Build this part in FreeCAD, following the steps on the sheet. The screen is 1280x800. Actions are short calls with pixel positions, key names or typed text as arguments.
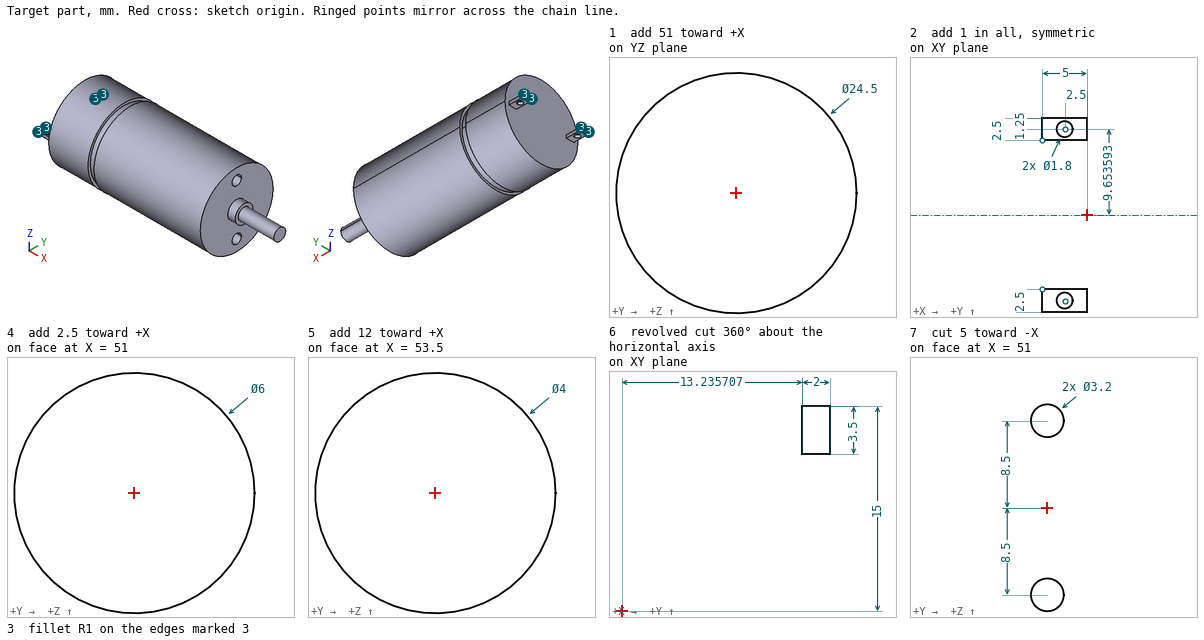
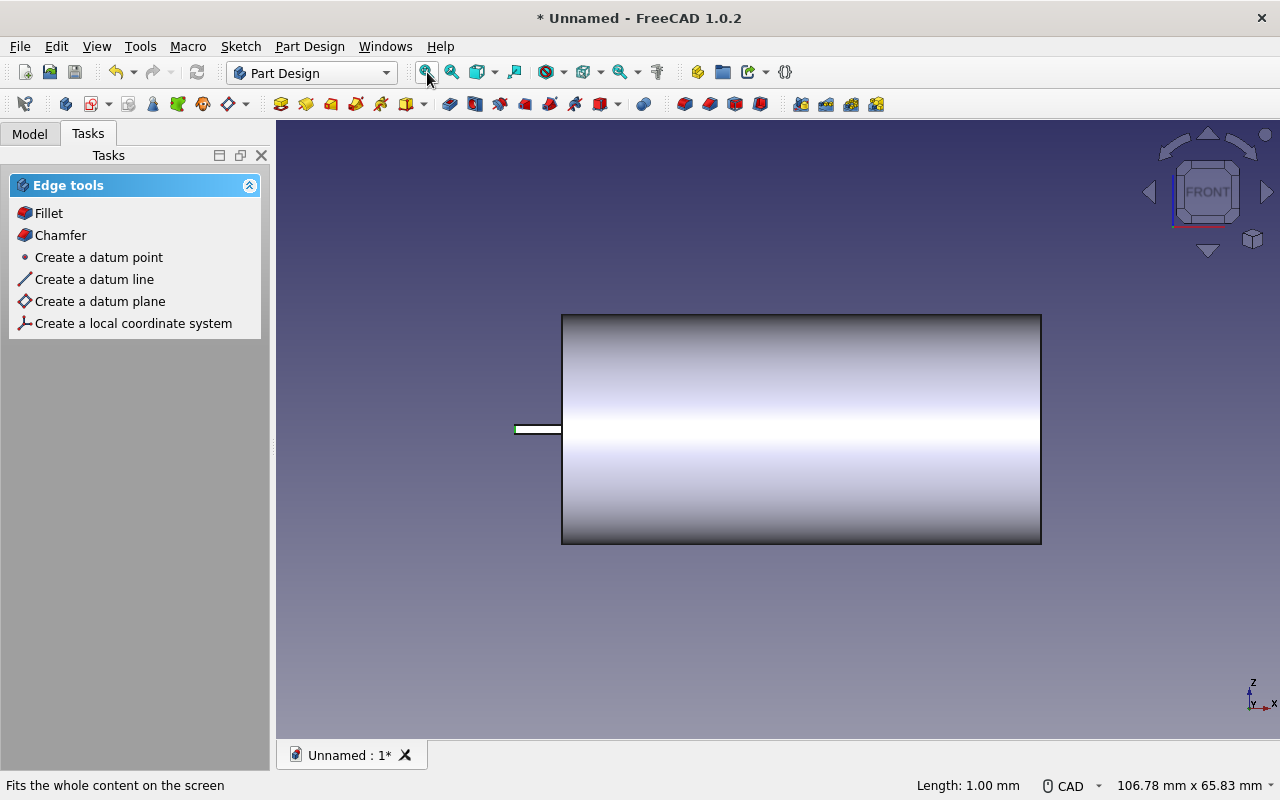
key(3)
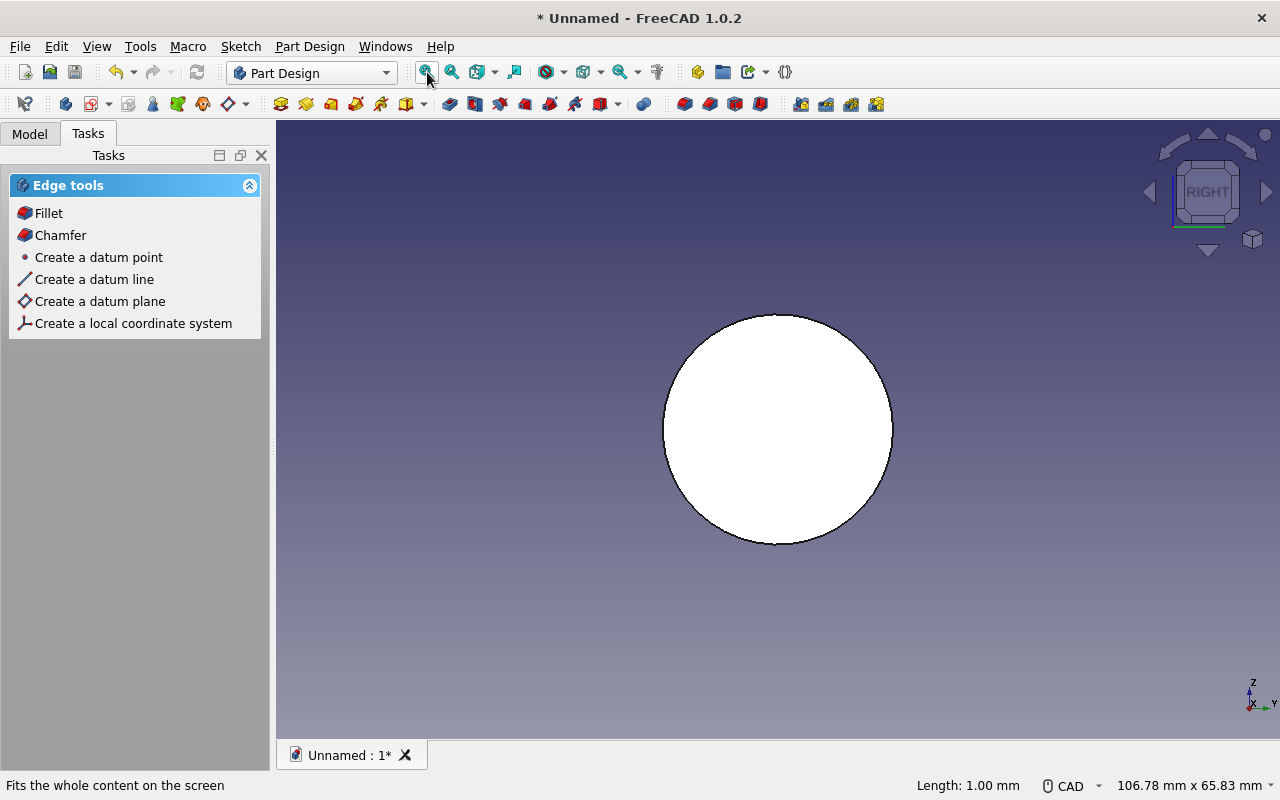
click(427, 72)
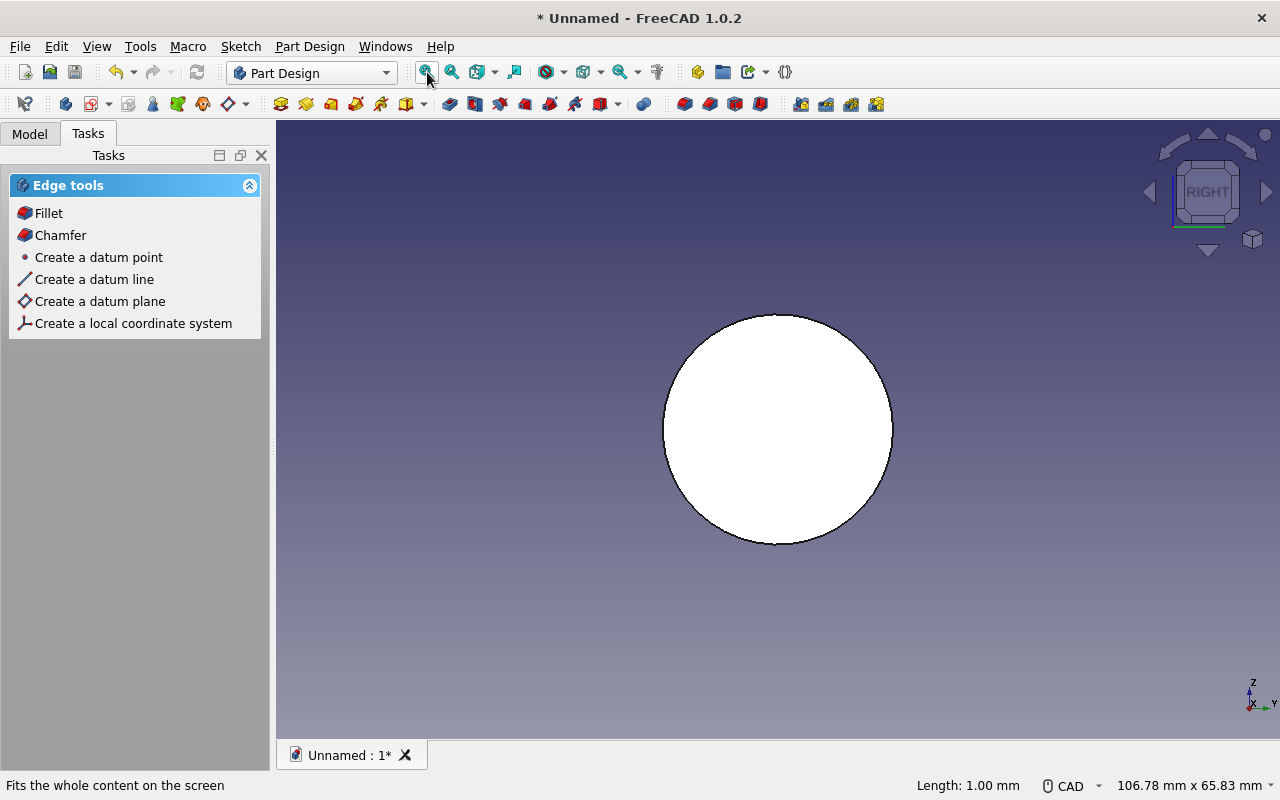
scroll(857, 428, up, 8)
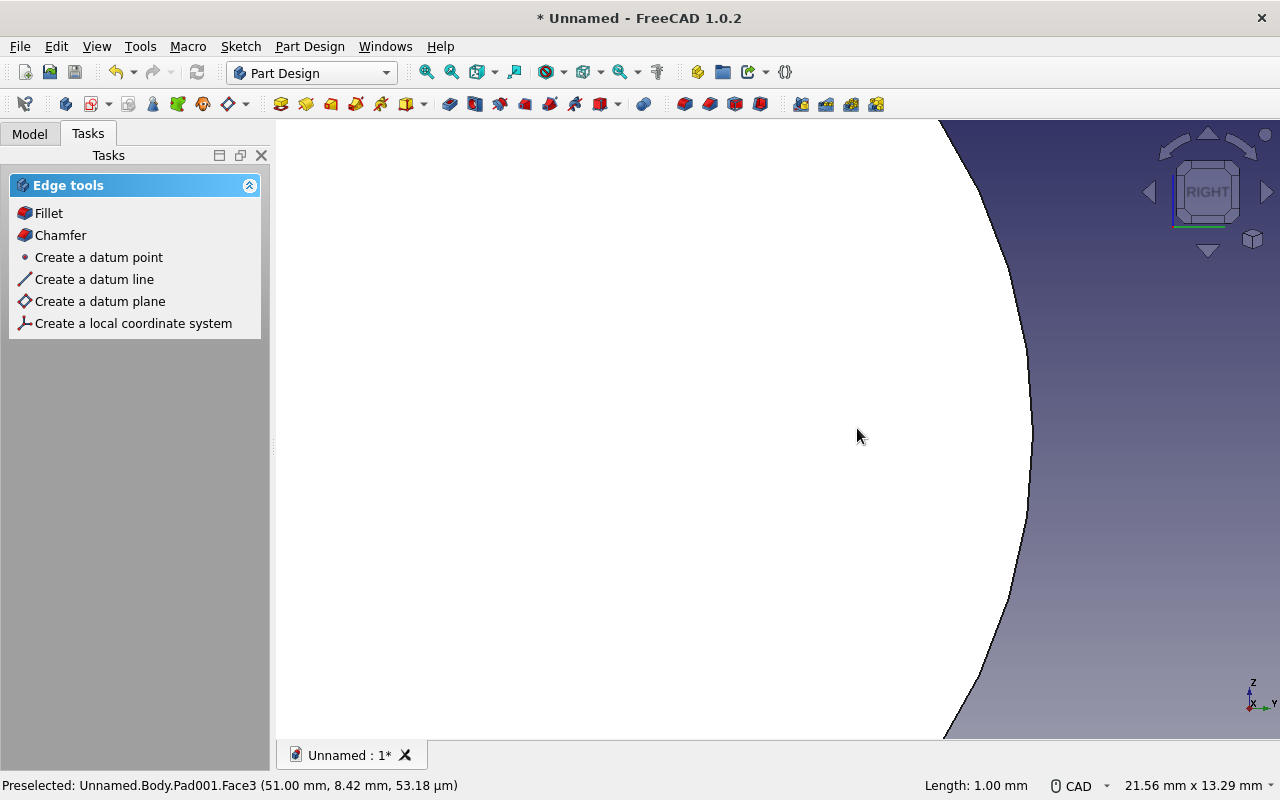
click(427, 72)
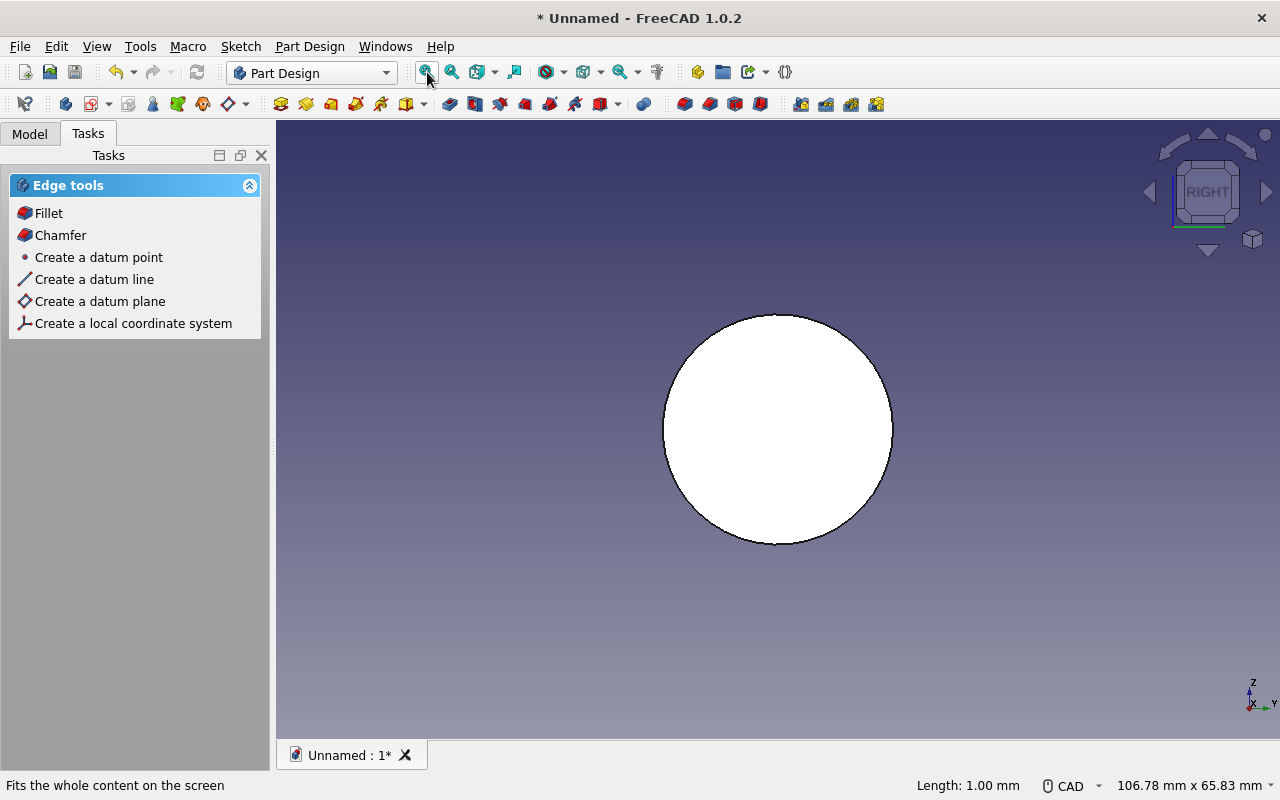
key(5)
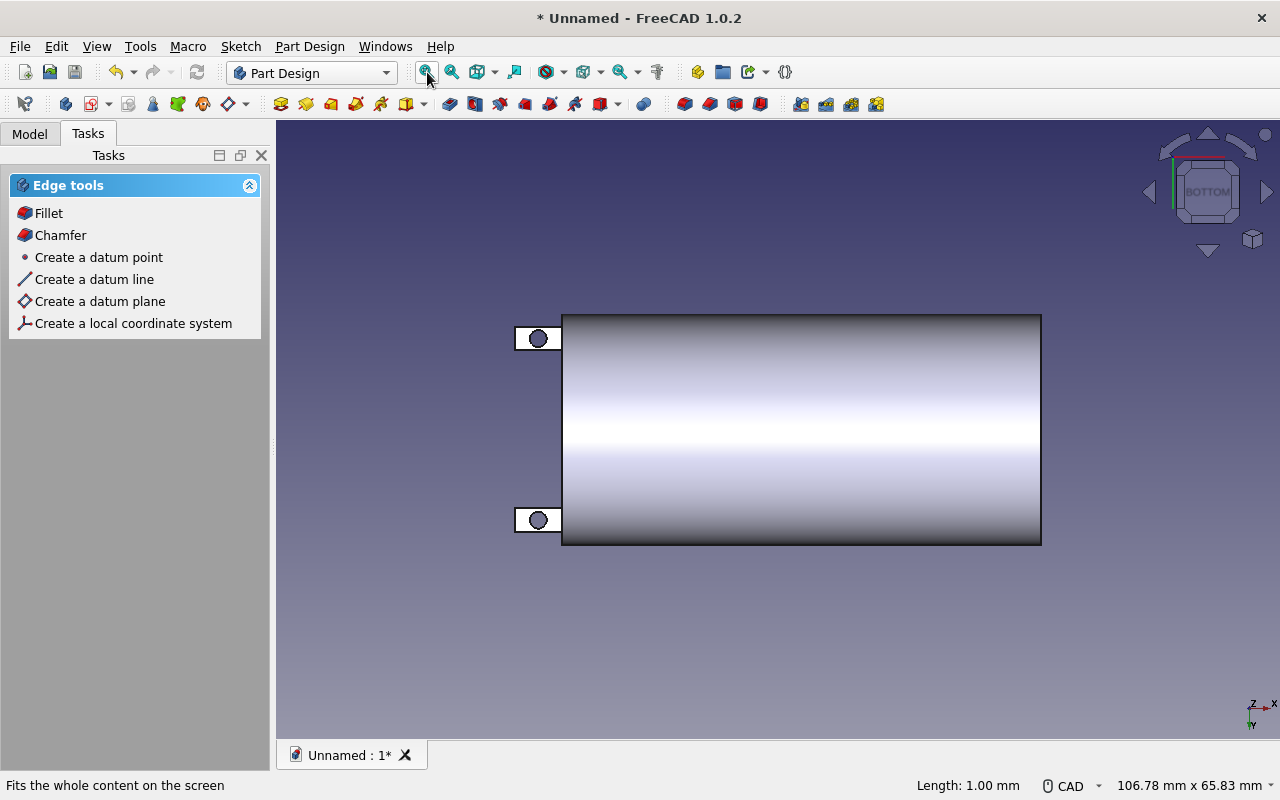
scroll(515, 507, up, 8)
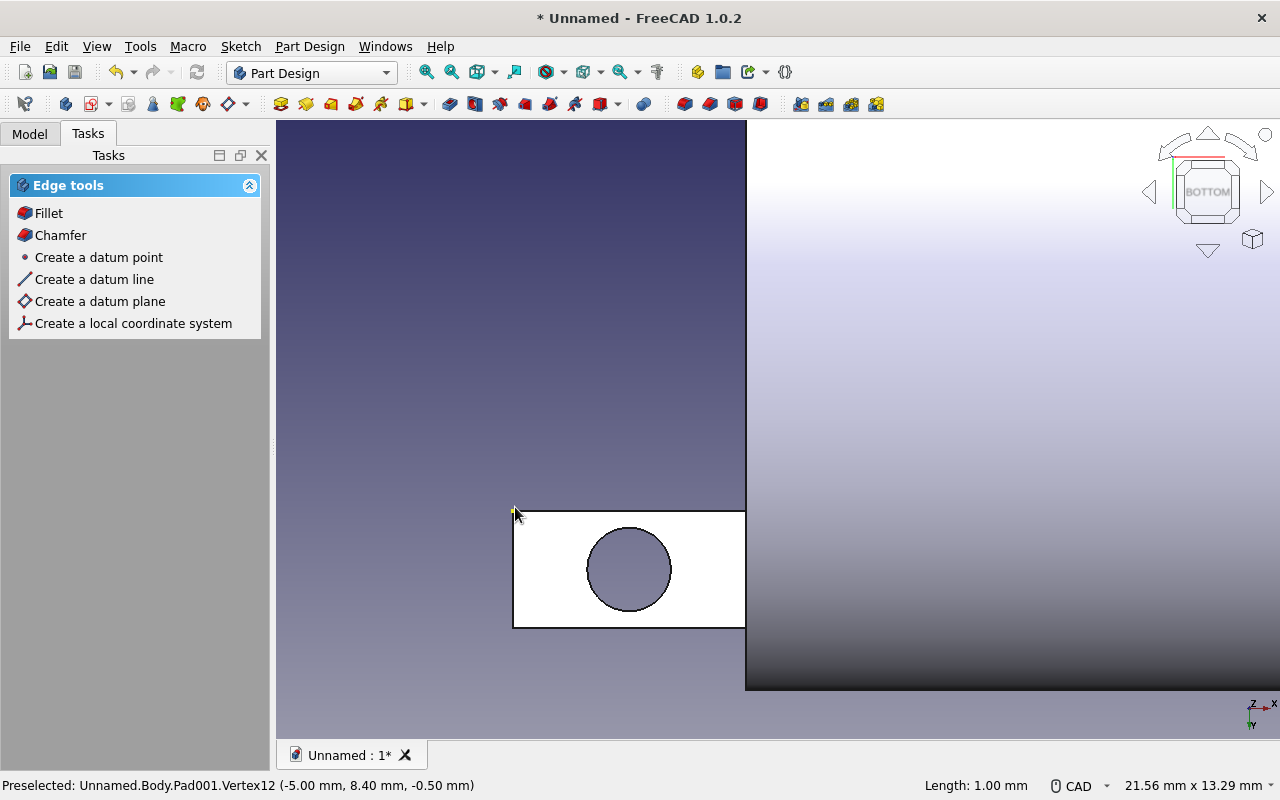
click(427, 72)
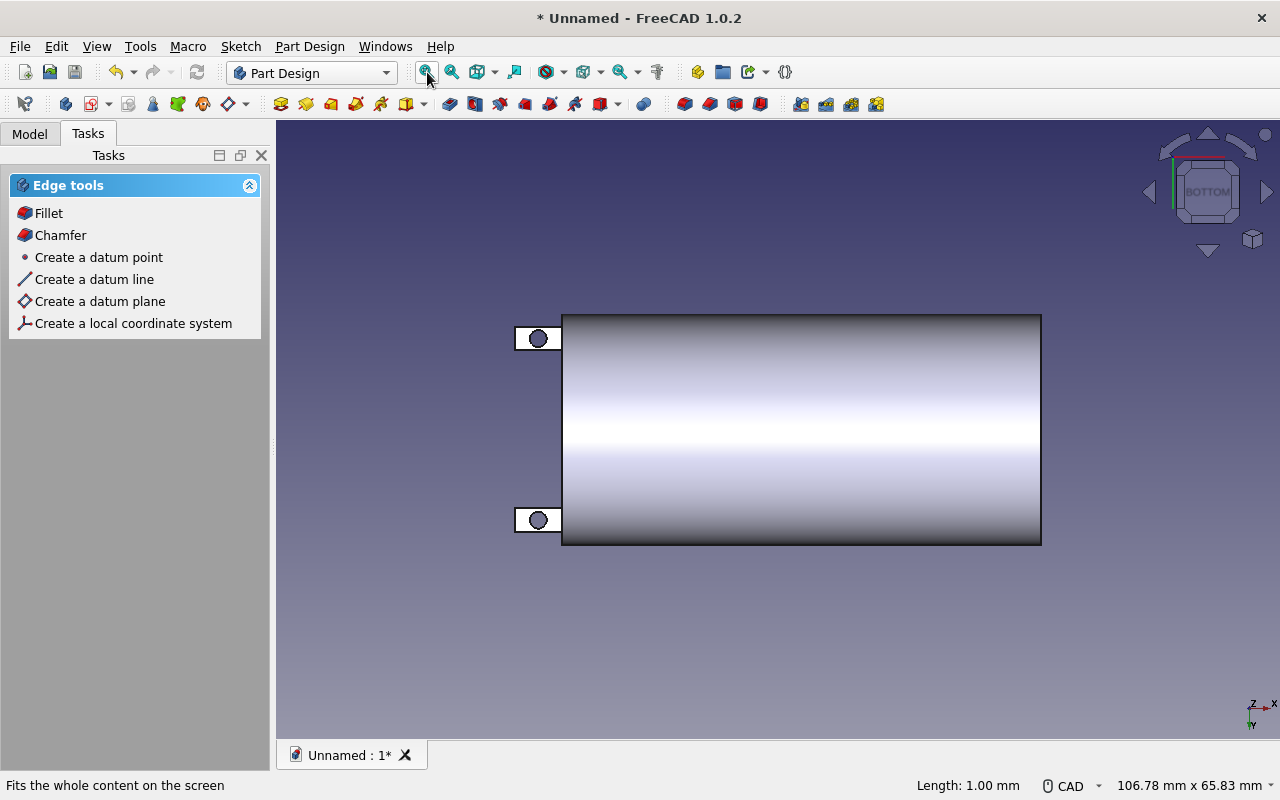
key(4)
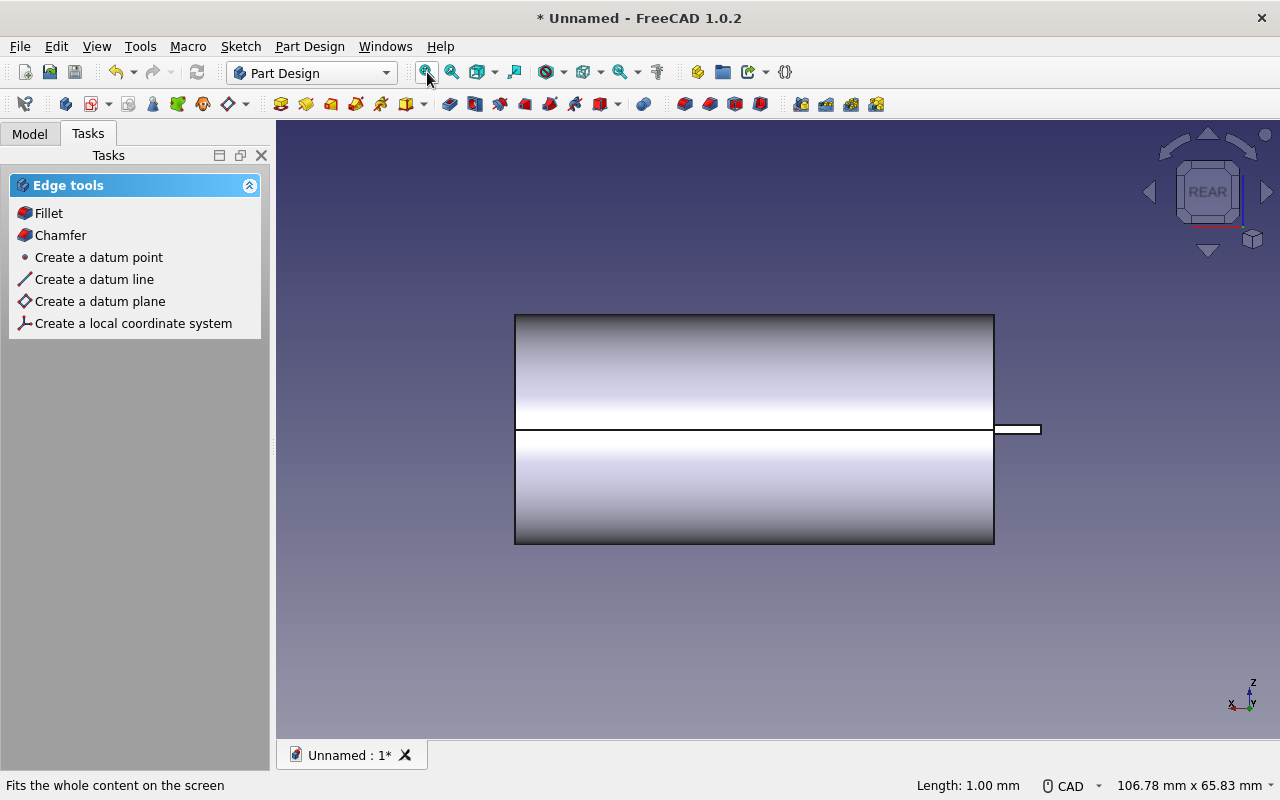
scroll(1041, 428, up, 8)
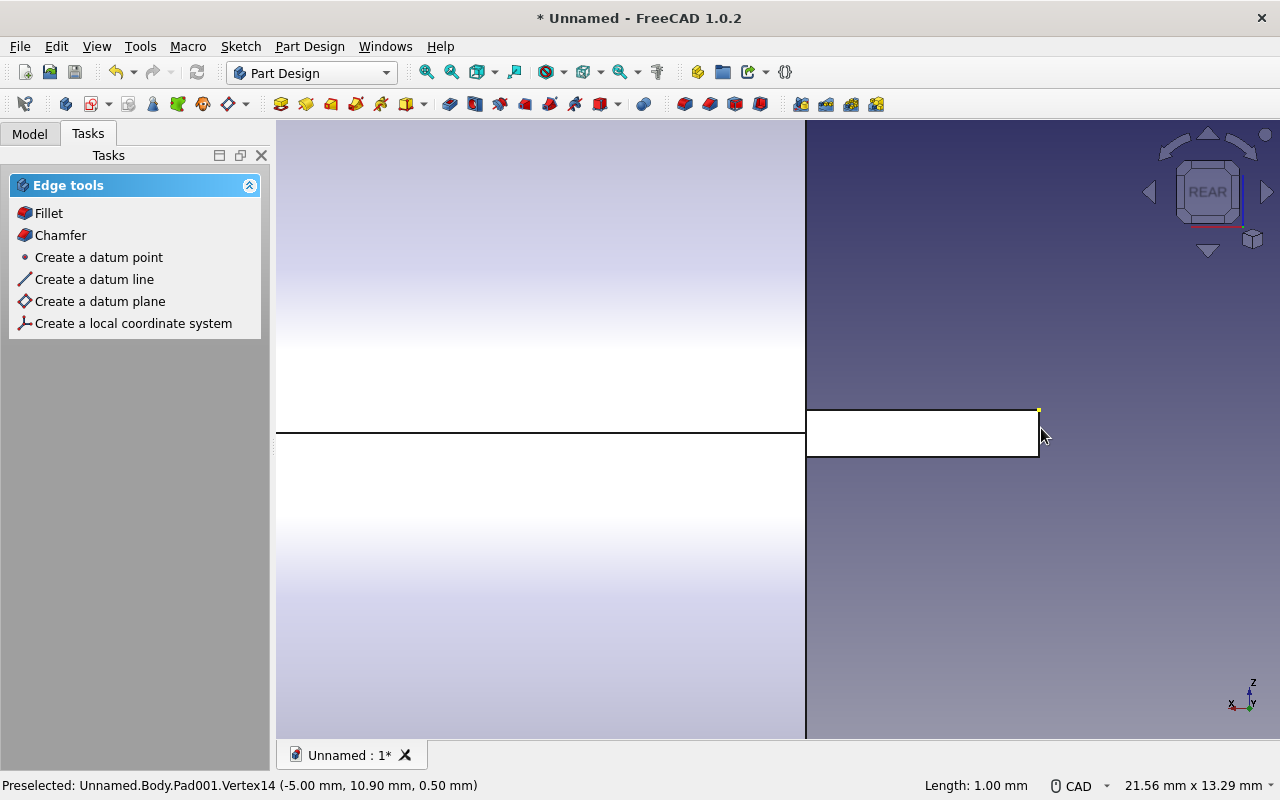
click(1039, 432, ctrl)